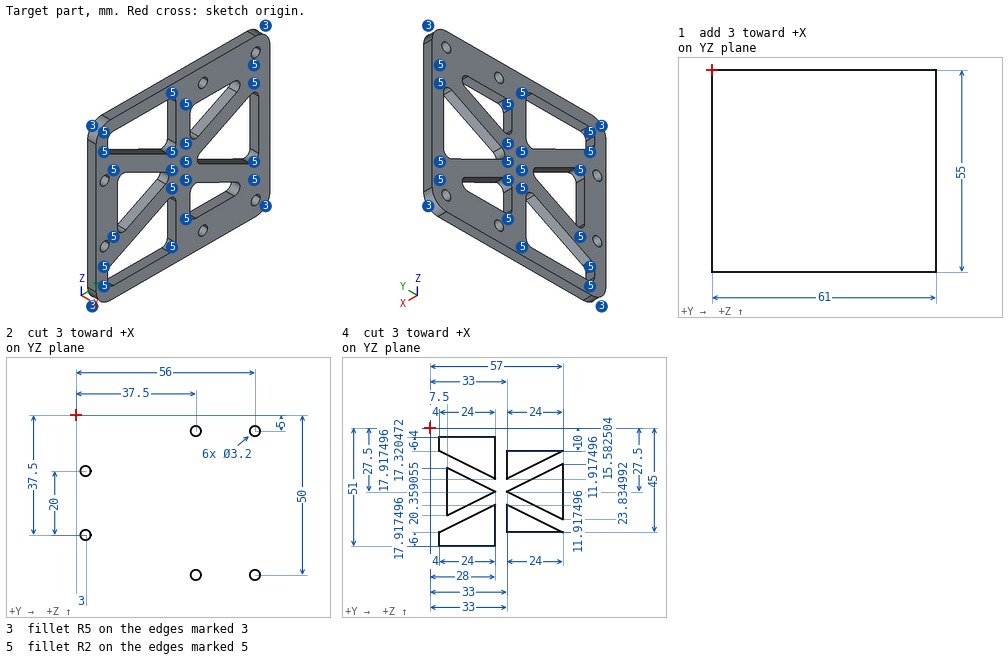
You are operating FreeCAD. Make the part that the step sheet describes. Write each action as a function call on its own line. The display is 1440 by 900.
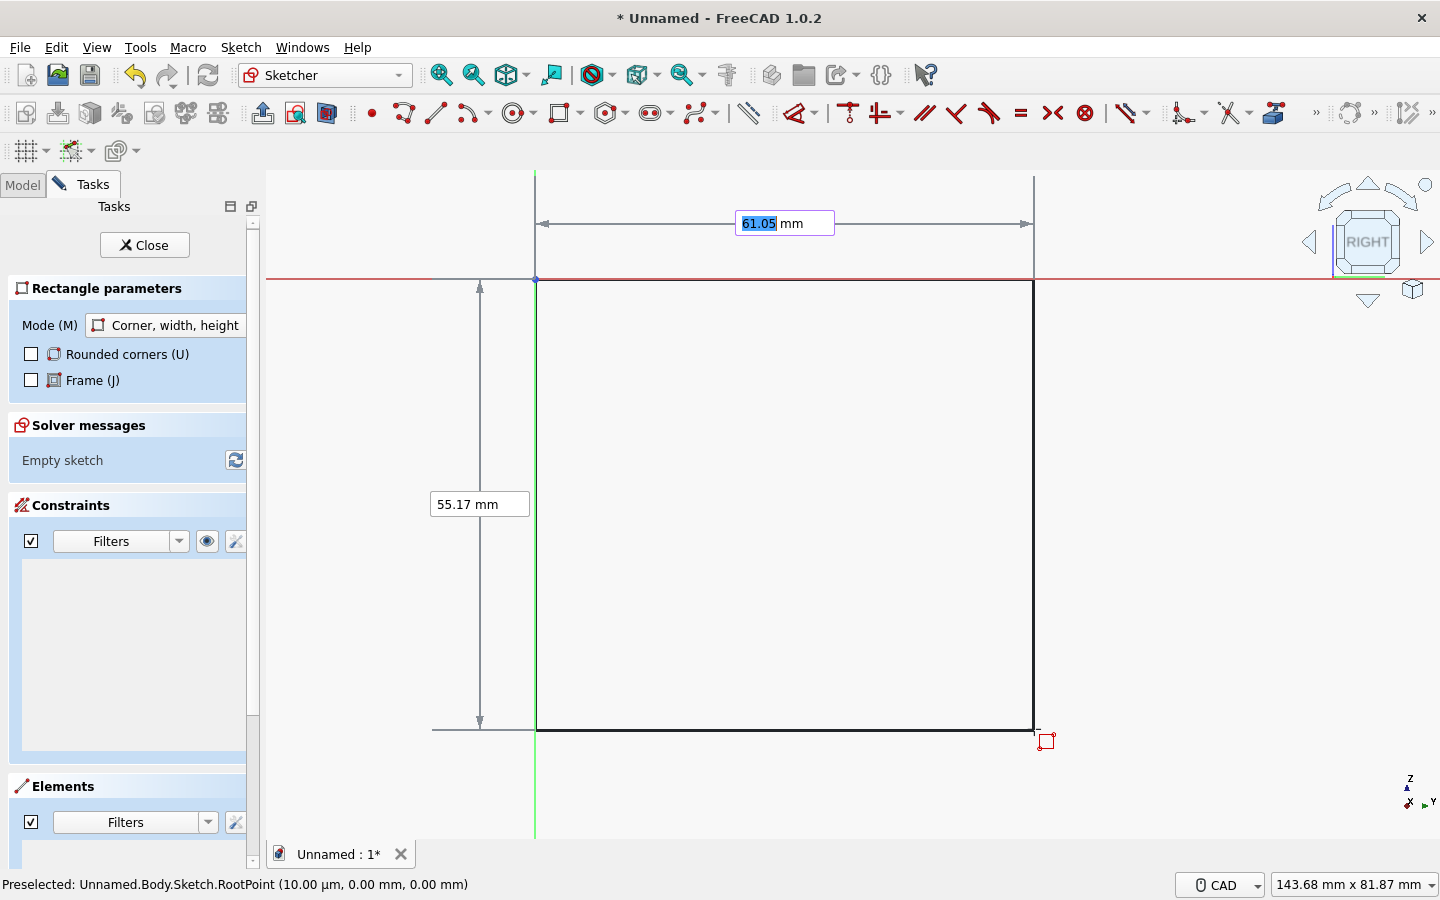
text(61)
key(Tab)
text(55)
key(Return)
key(Escape)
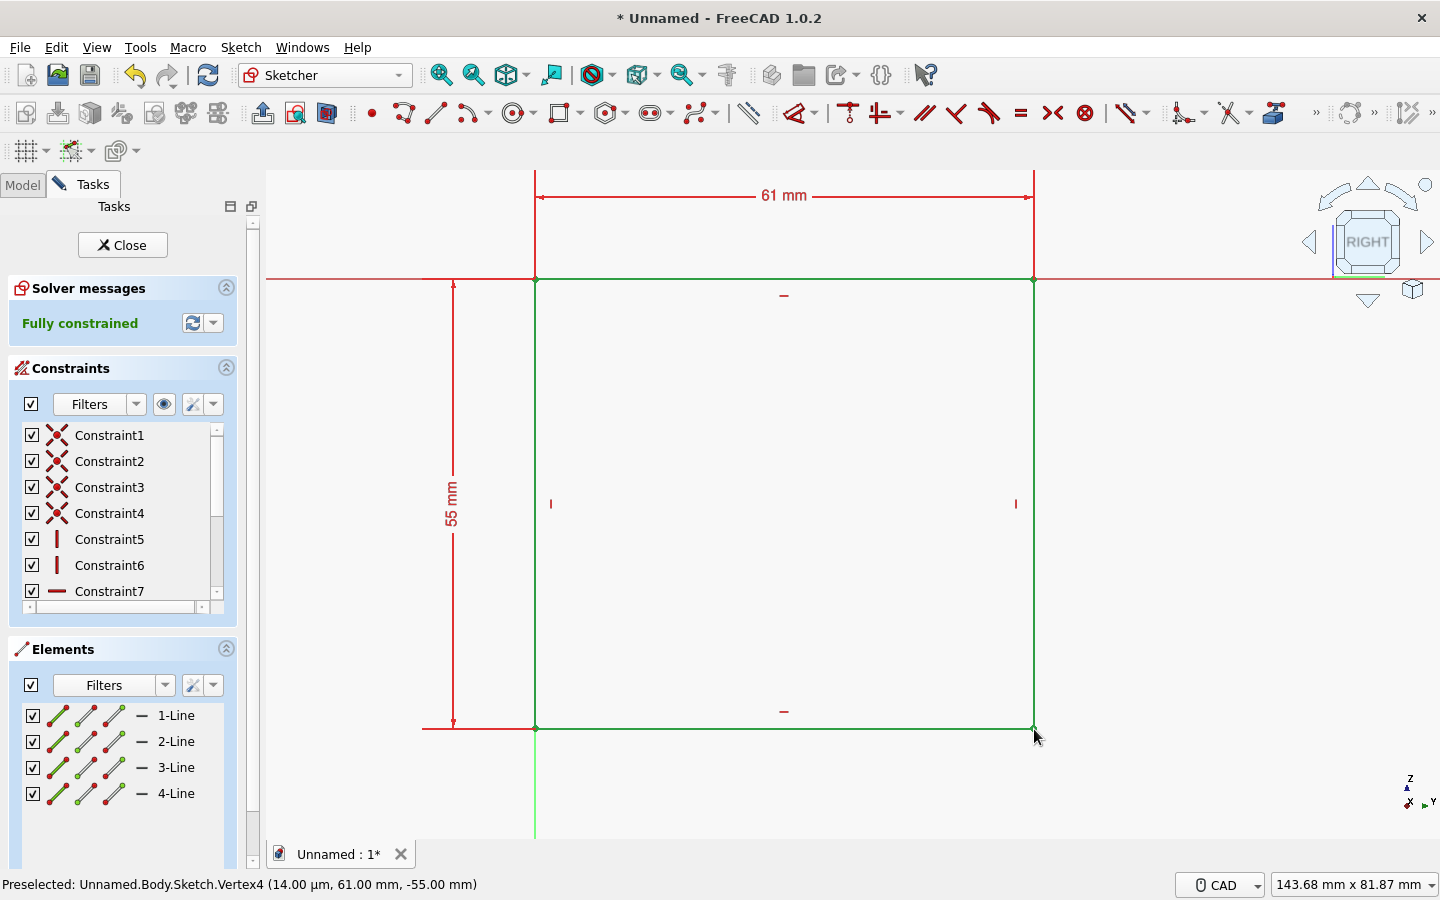
click(123, 245)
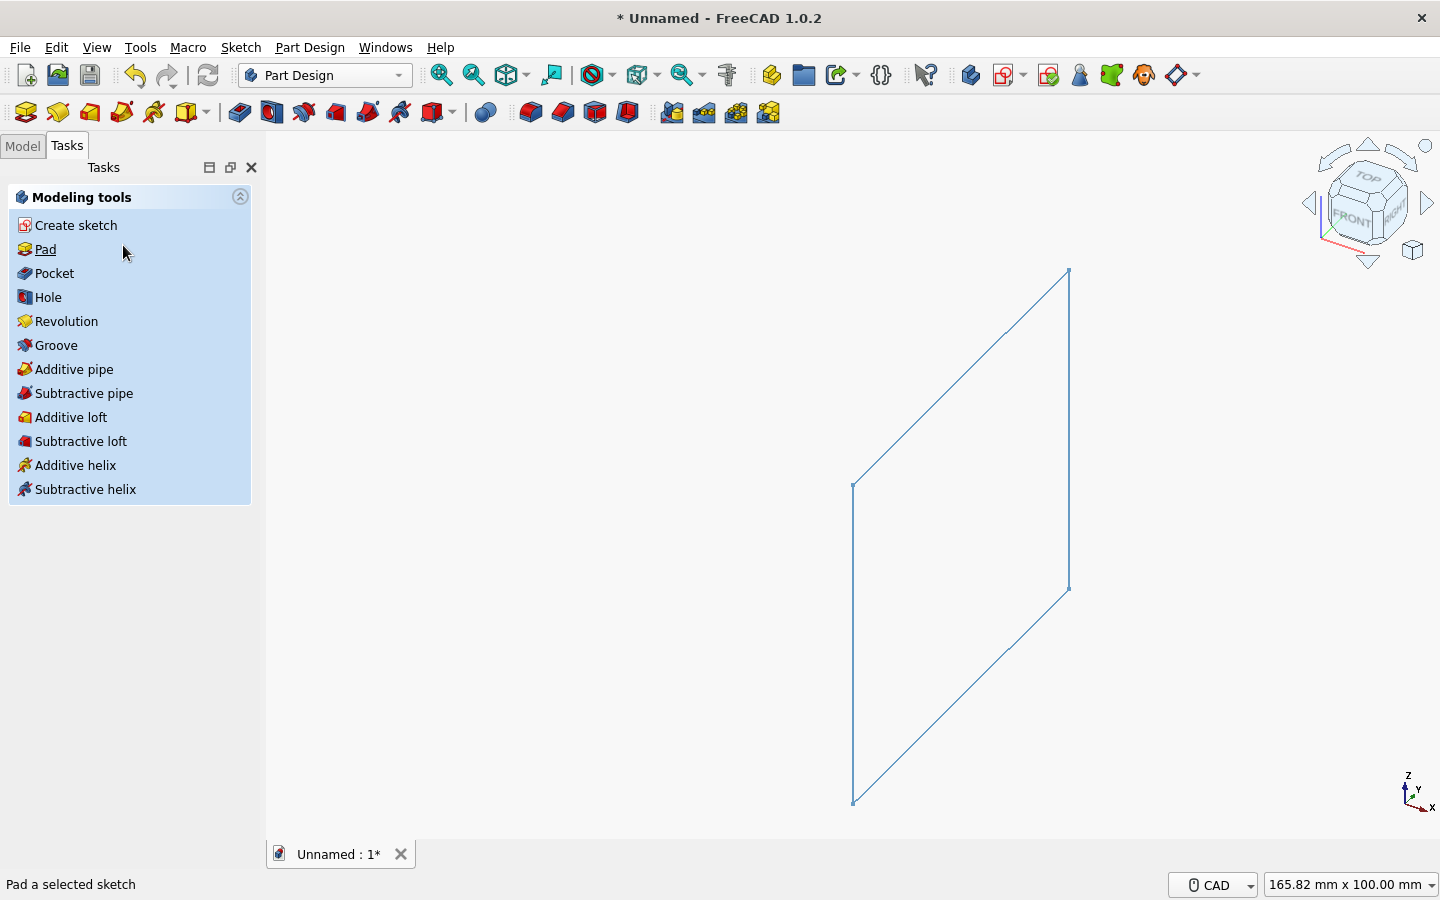
click(26, 112)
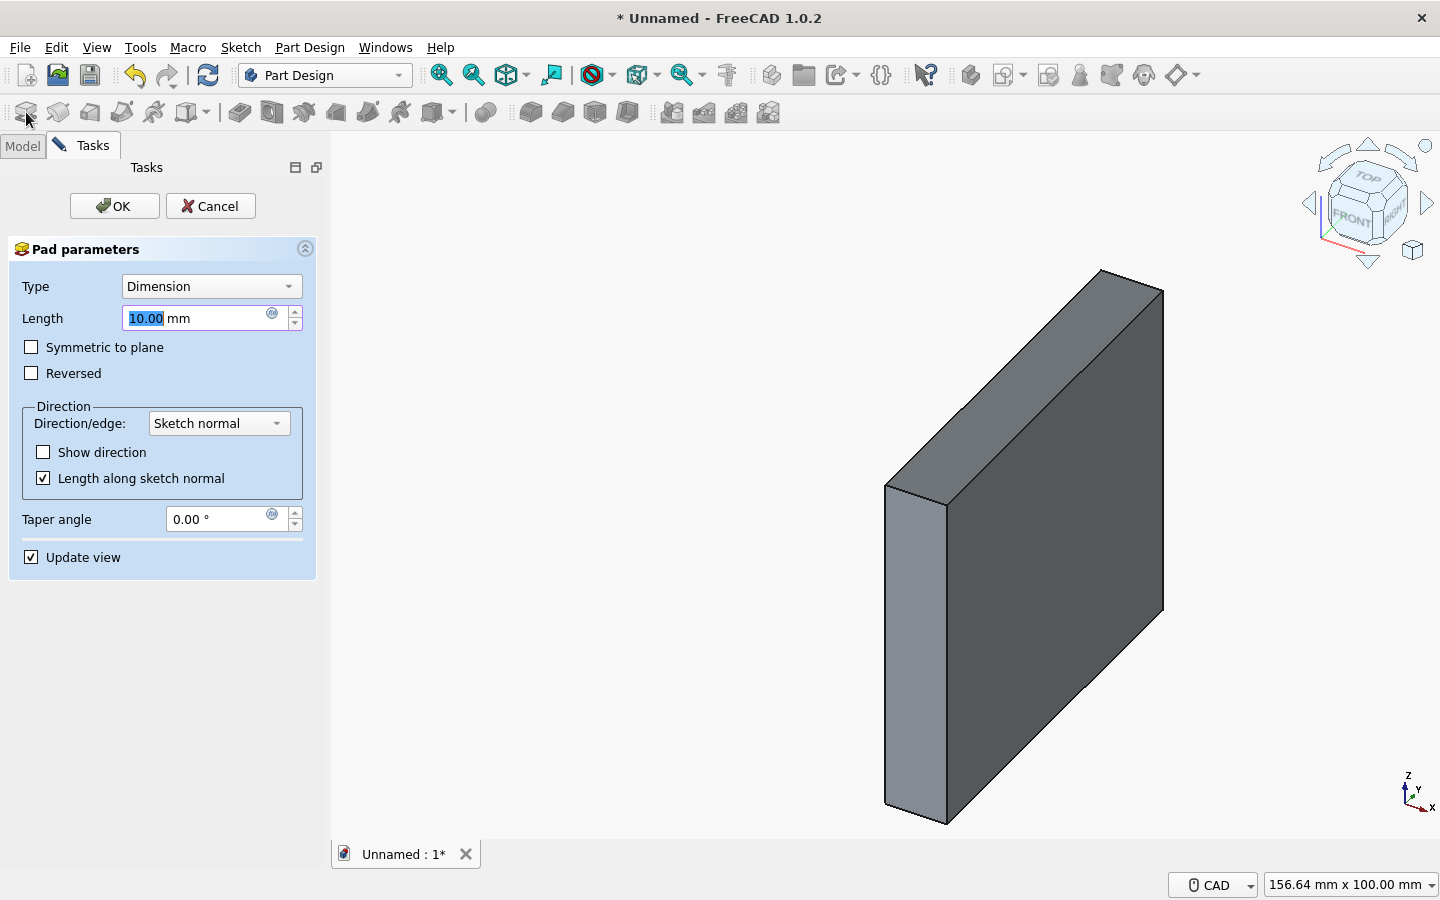
text(3)
key(Tab)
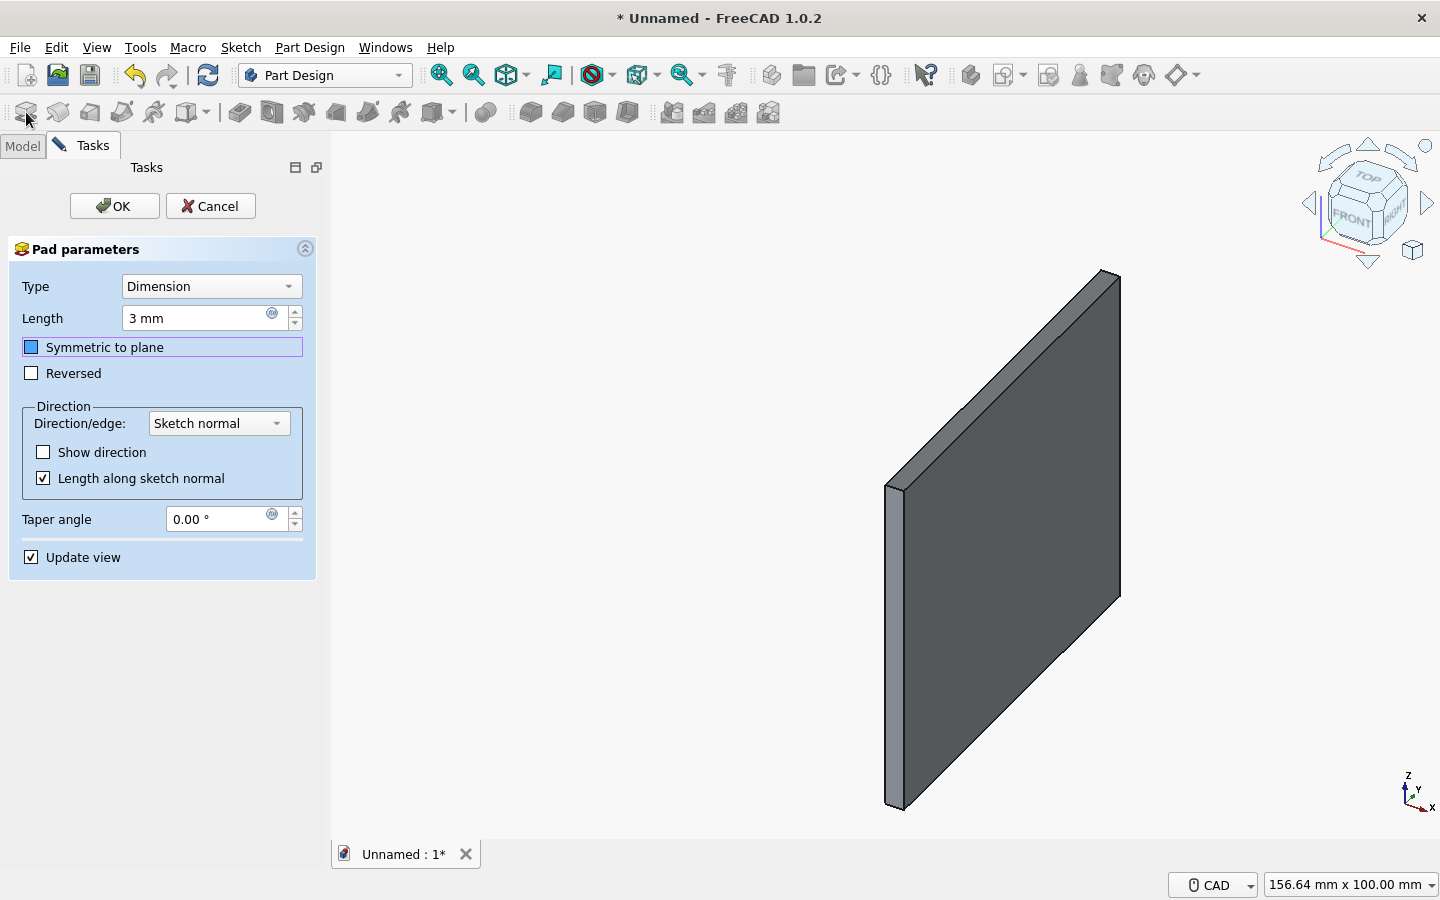
click(115, 206)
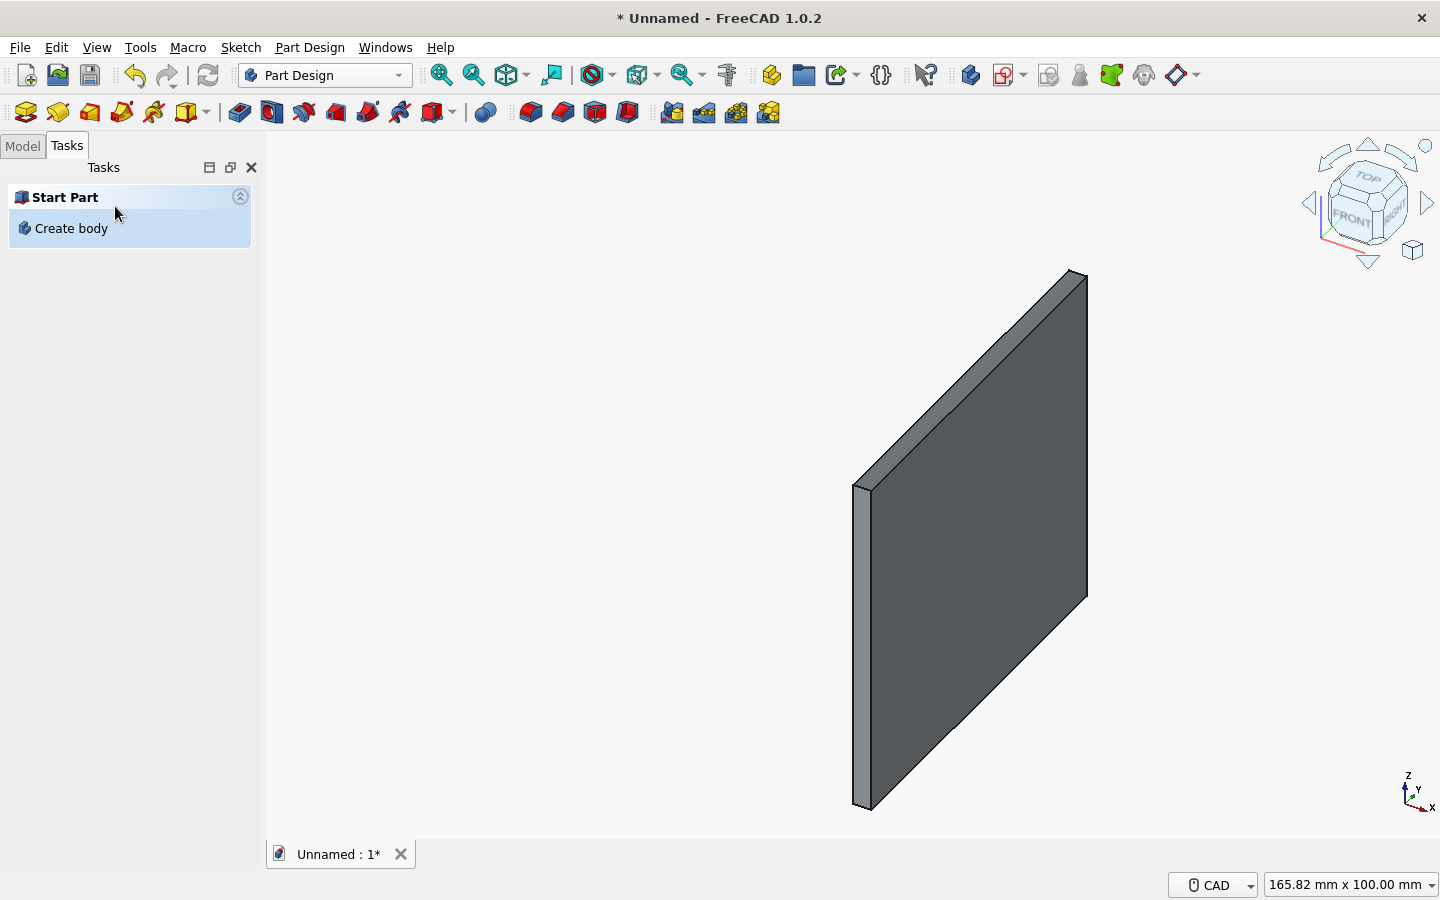
click(1004, 76)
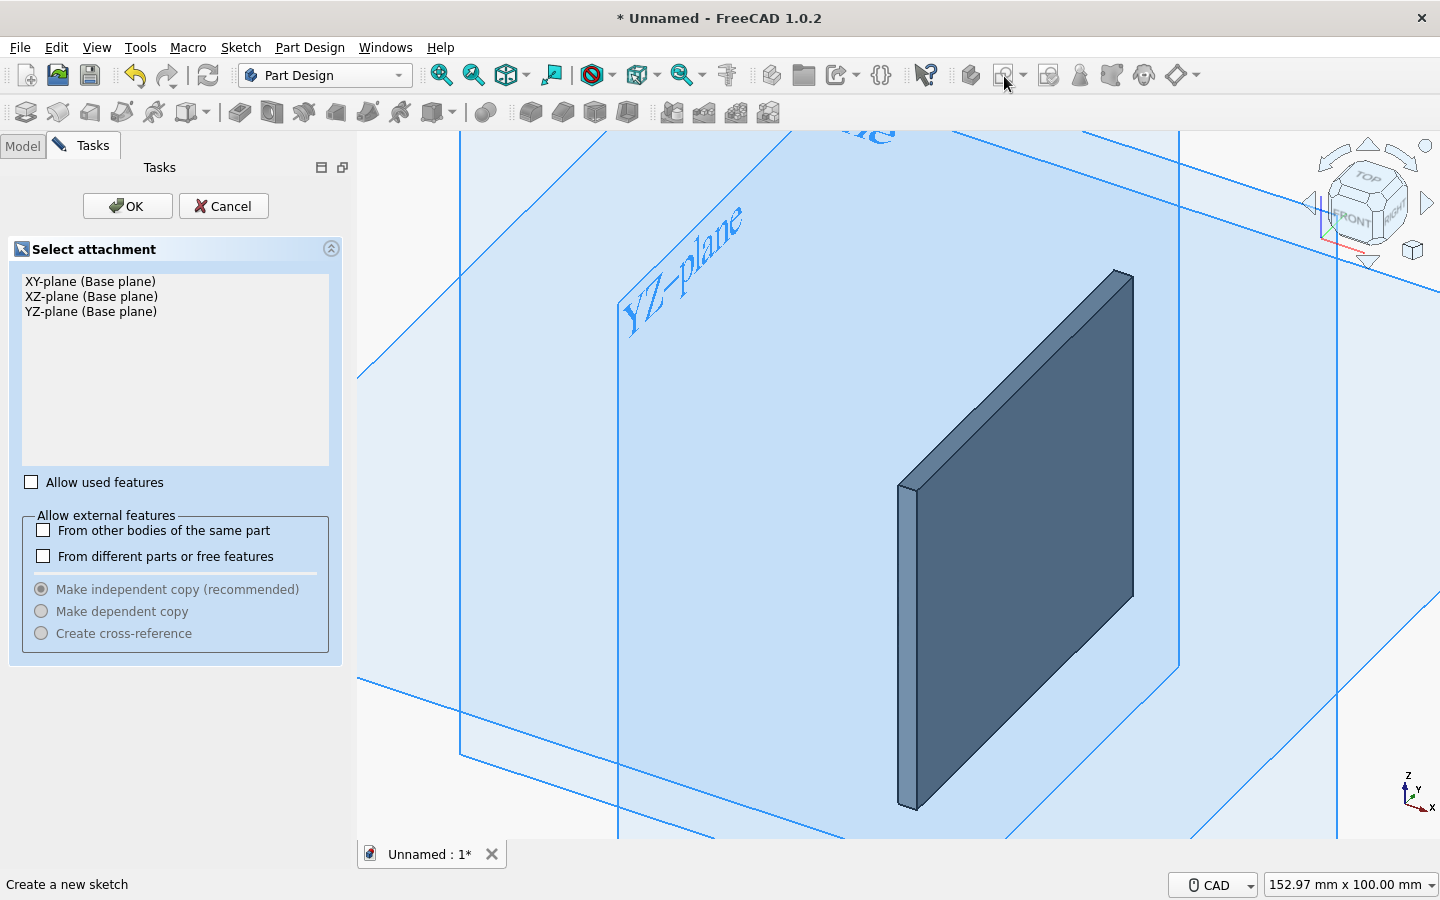
click(82, 312)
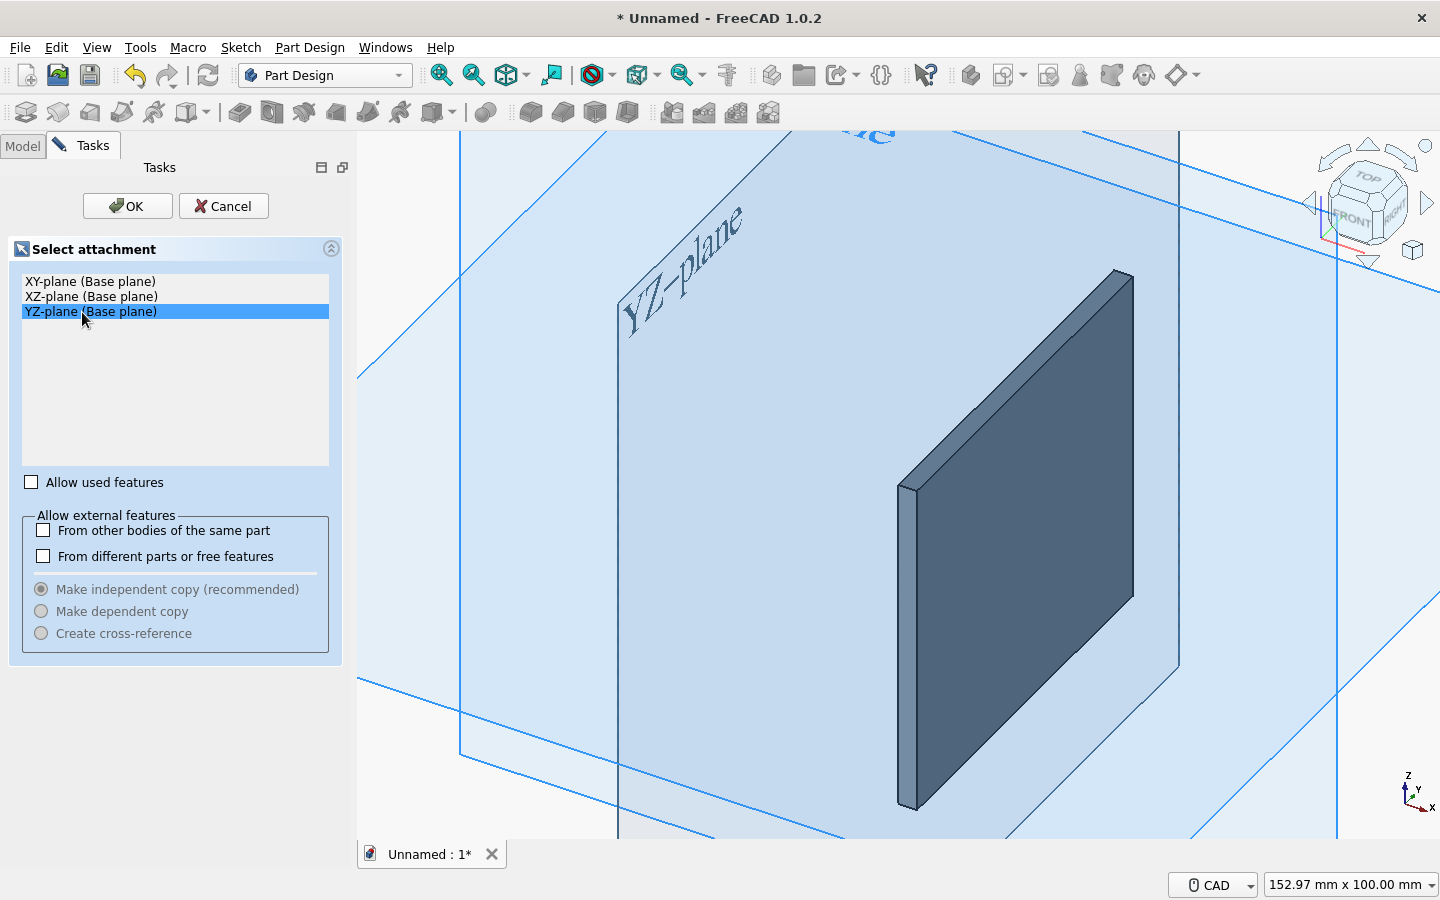
click(128, 206)